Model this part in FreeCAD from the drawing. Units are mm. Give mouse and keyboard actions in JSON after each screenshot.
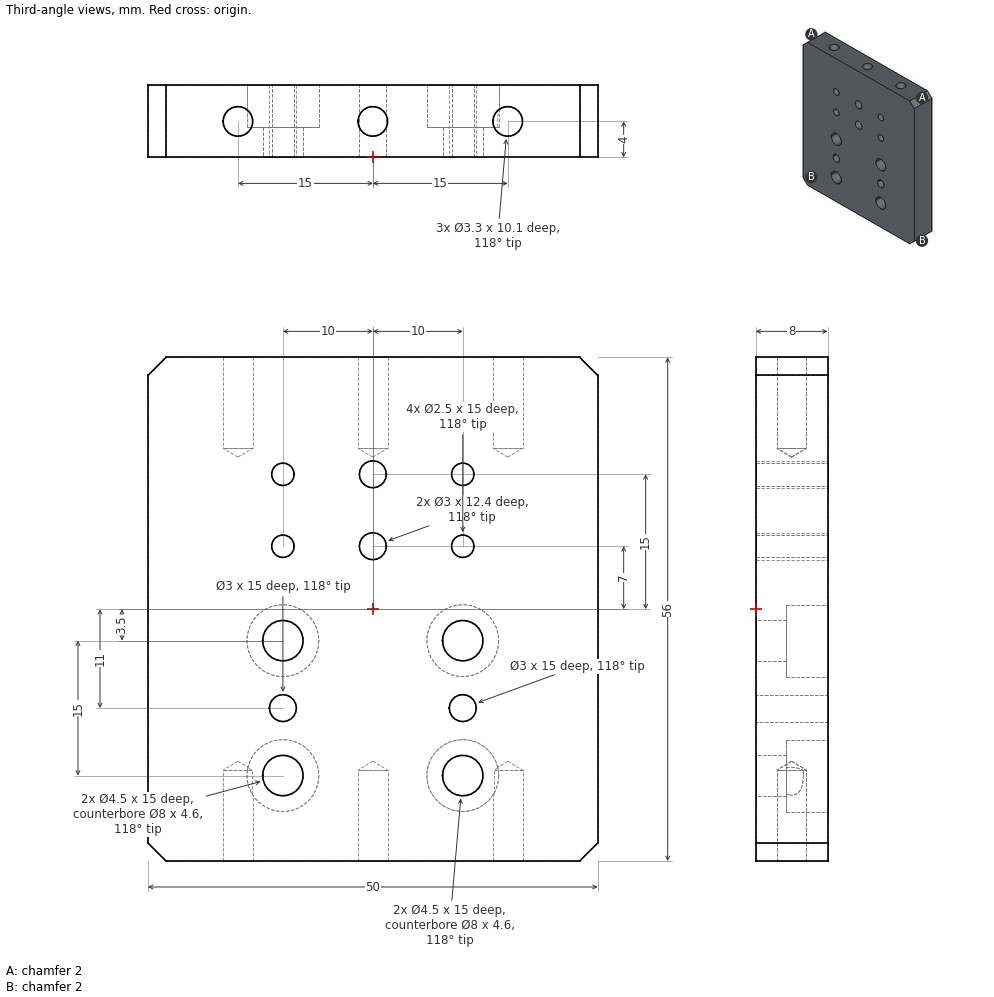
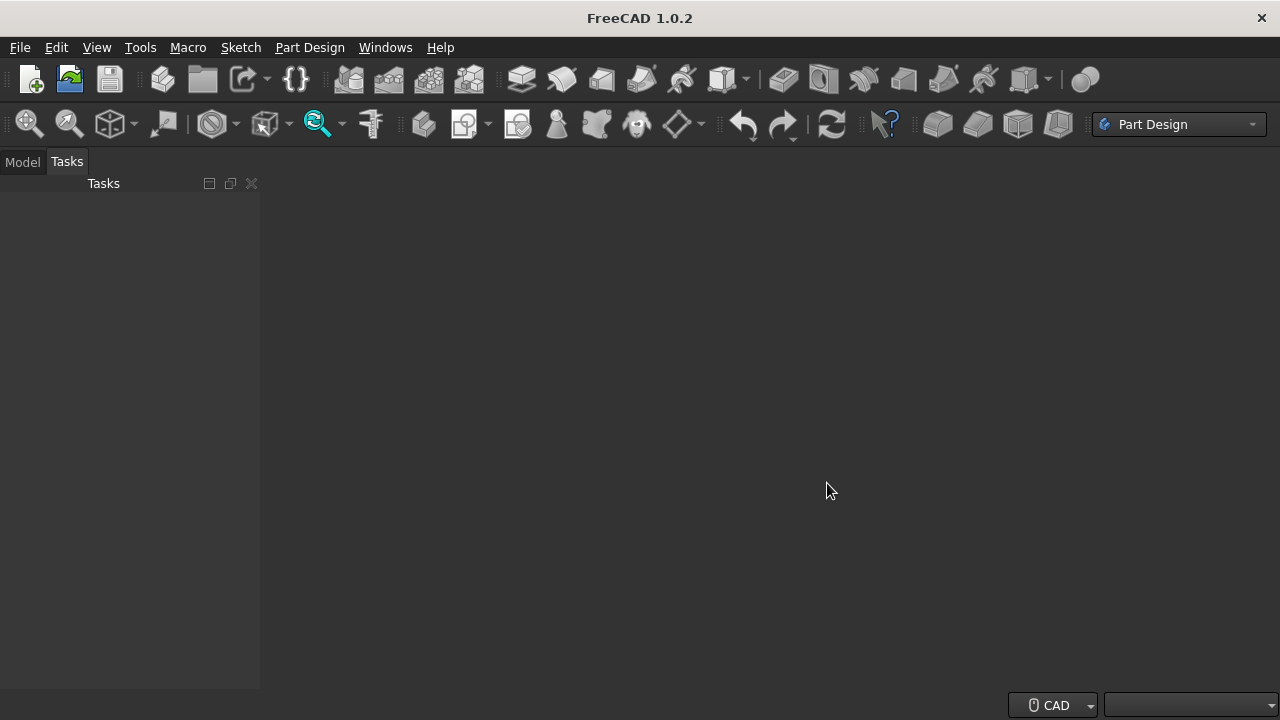
{"action": "left_click", "coordinate": [30, 80]}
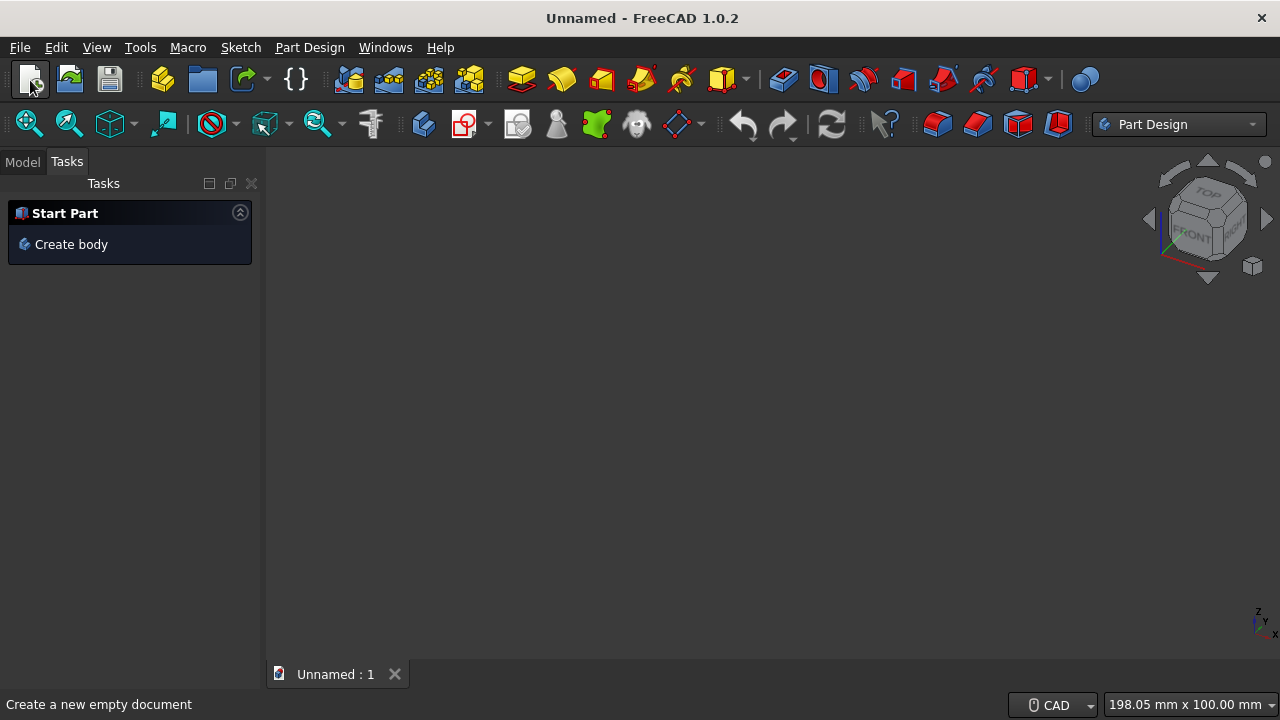
{"action": "left_click", "coordinate": [464, 124]}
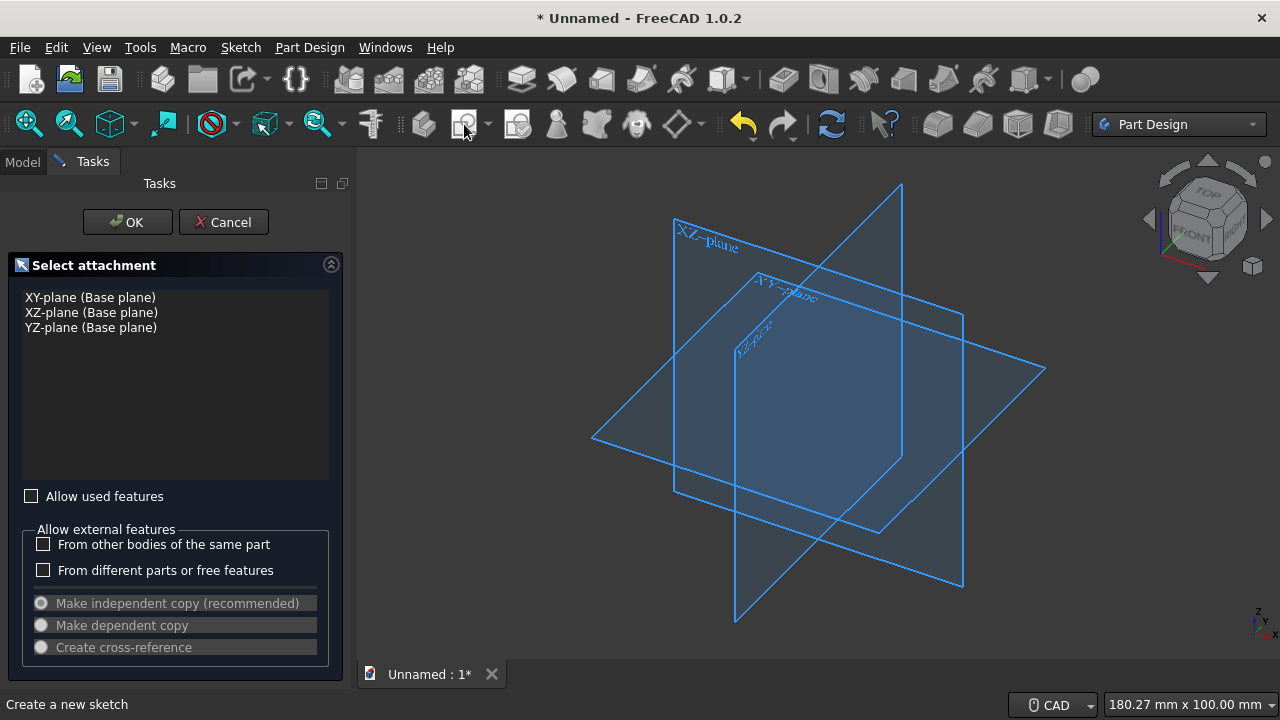
{"action": "left_click", "coordinate": [82, 312]}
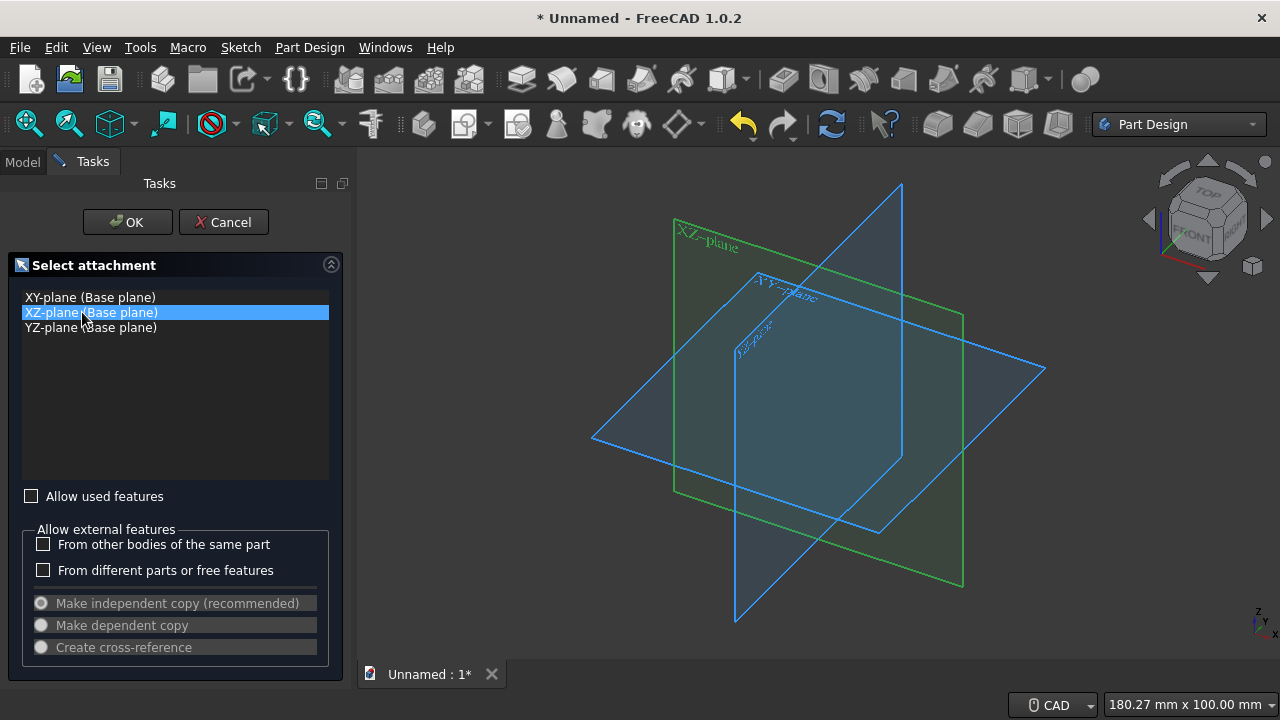
{"action": "left_click", "coordinate": [128, 222]}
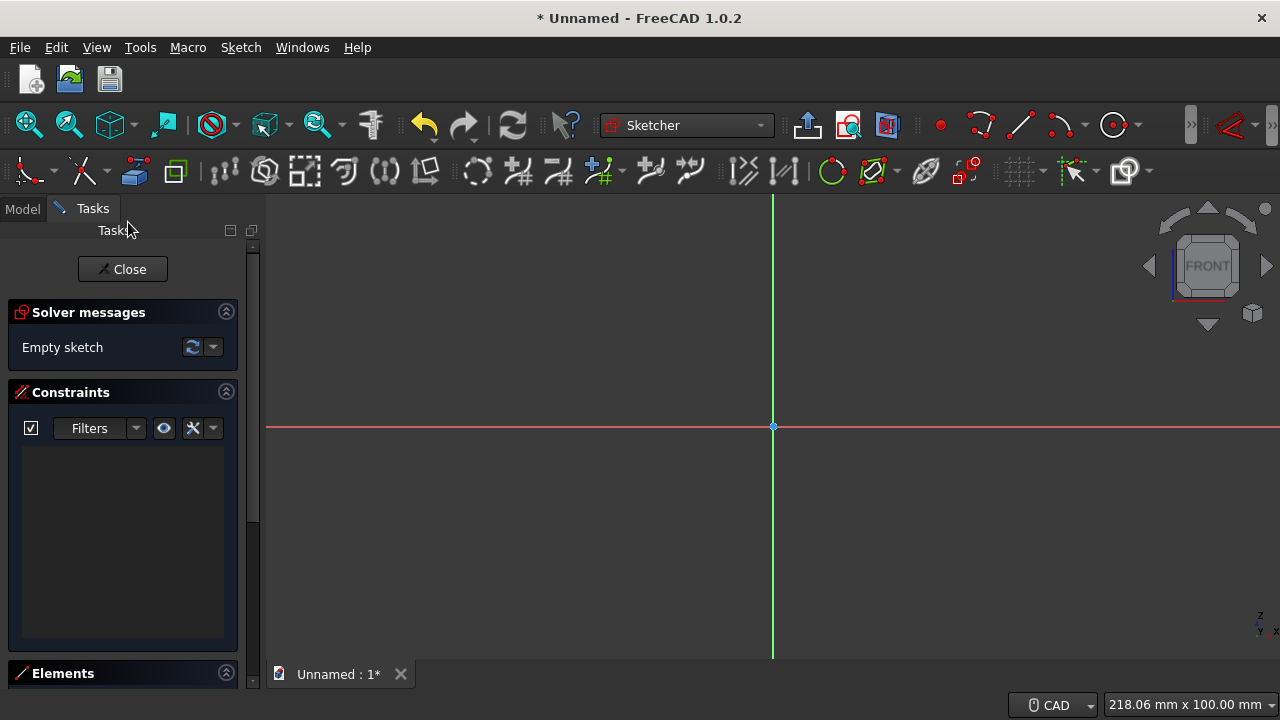
{"action": "key", "text": "g v"}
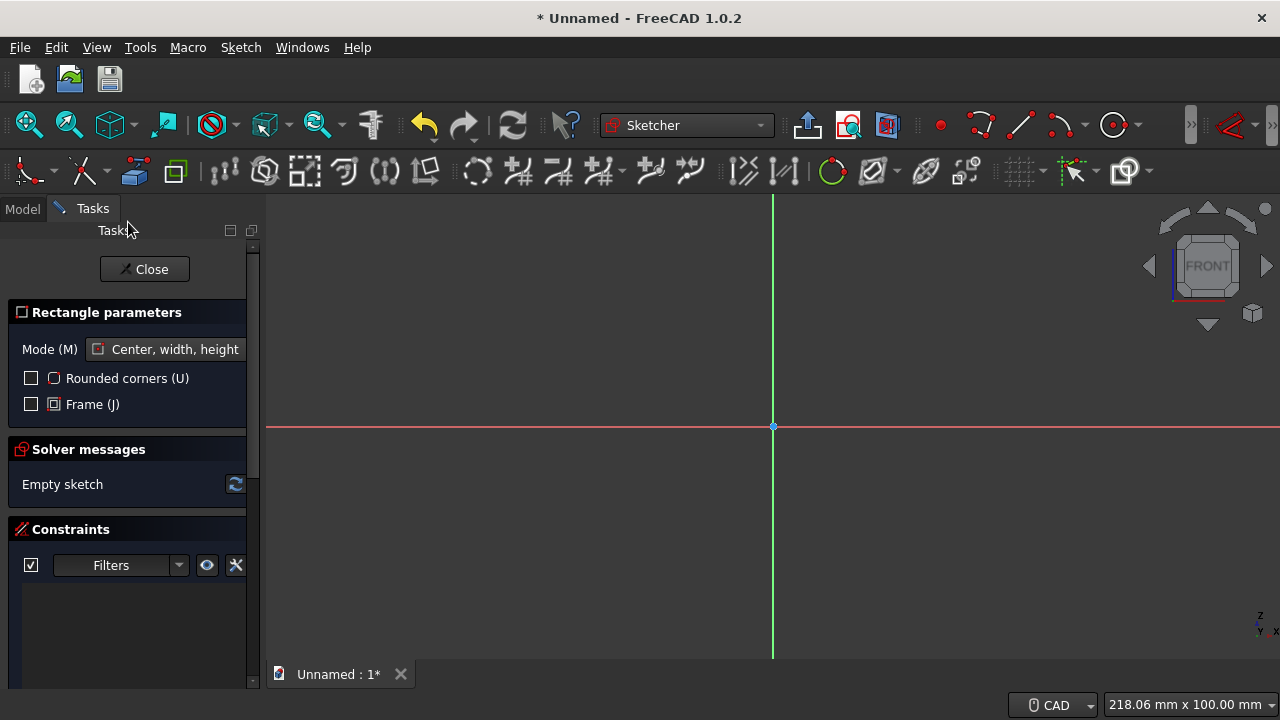
{"action": "left_click", "coordinate": [773, 426]}
{"action": "mouse_move", "coordinate": [889, 296]}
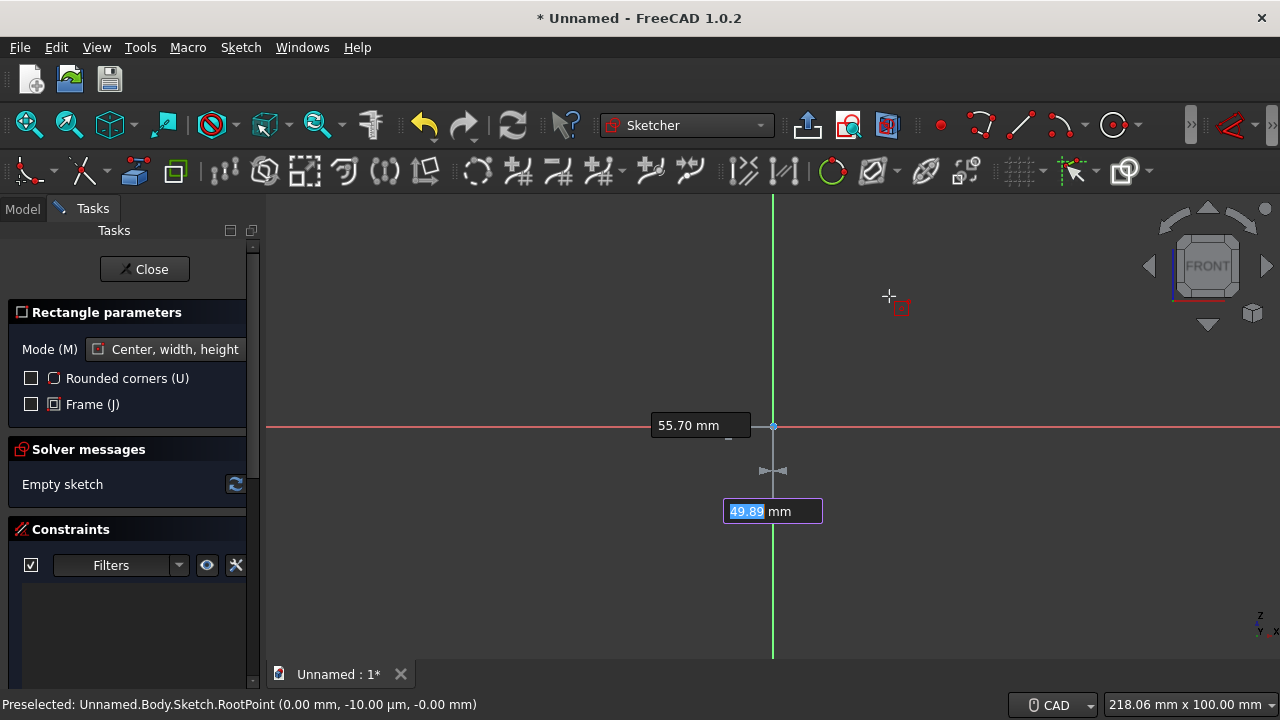
{"action": "type", "text": "50"}
{"action": "key", "text": "Tab"}
{"action": "type", "text": "56"}
{"action": "key", "text": "Return"}
{"action": "key", "text": "Escape"}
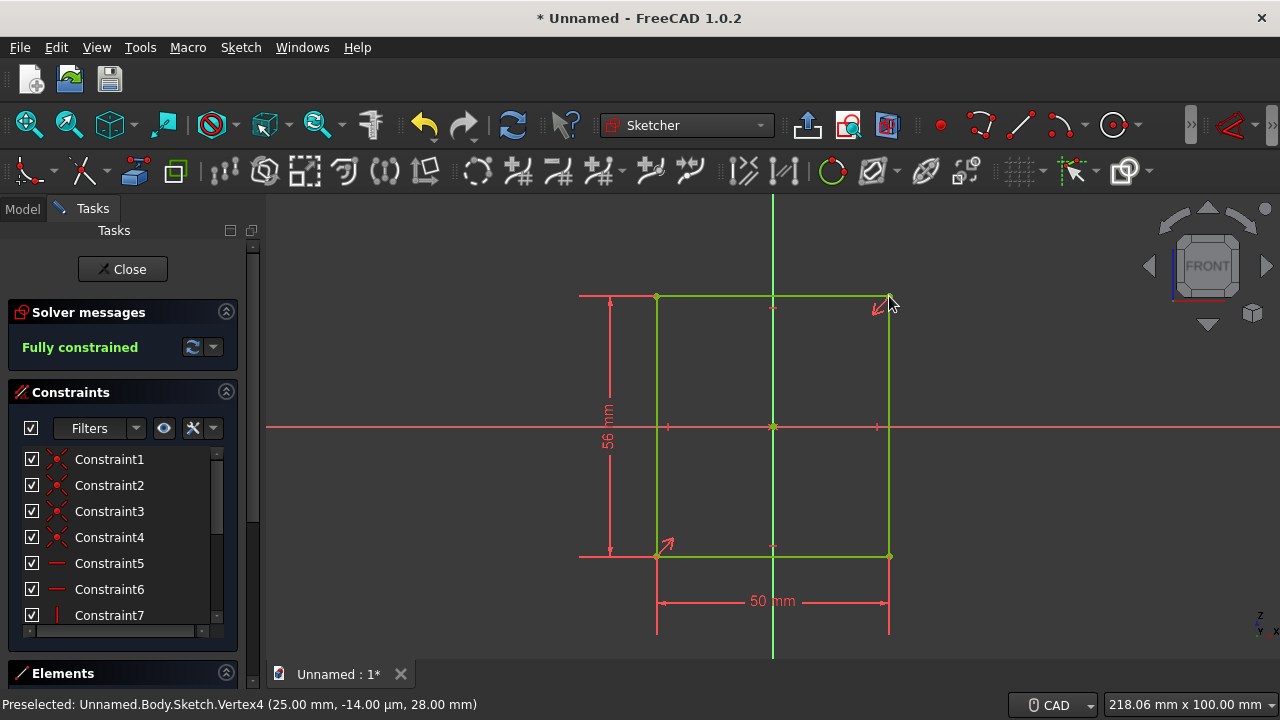
{"action": "left_click", "coordinate": [123, 269]}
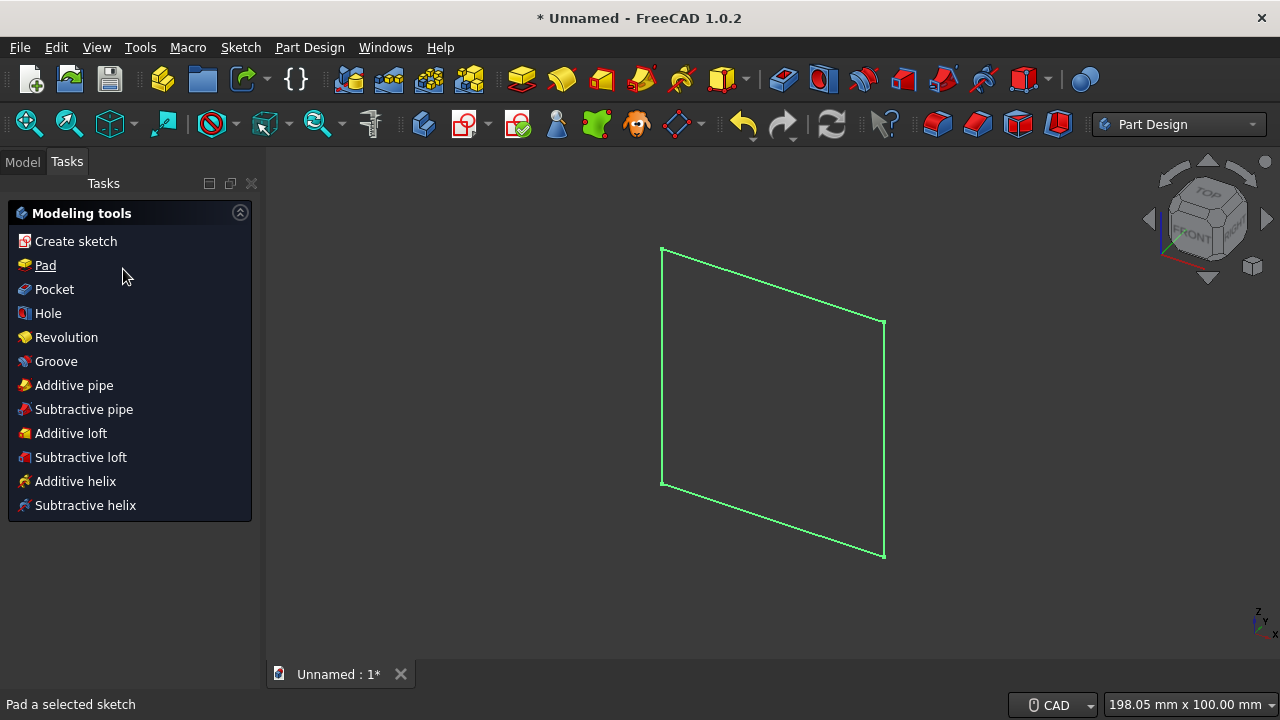
{"action": "left_click", "coordinate": [522, 80]}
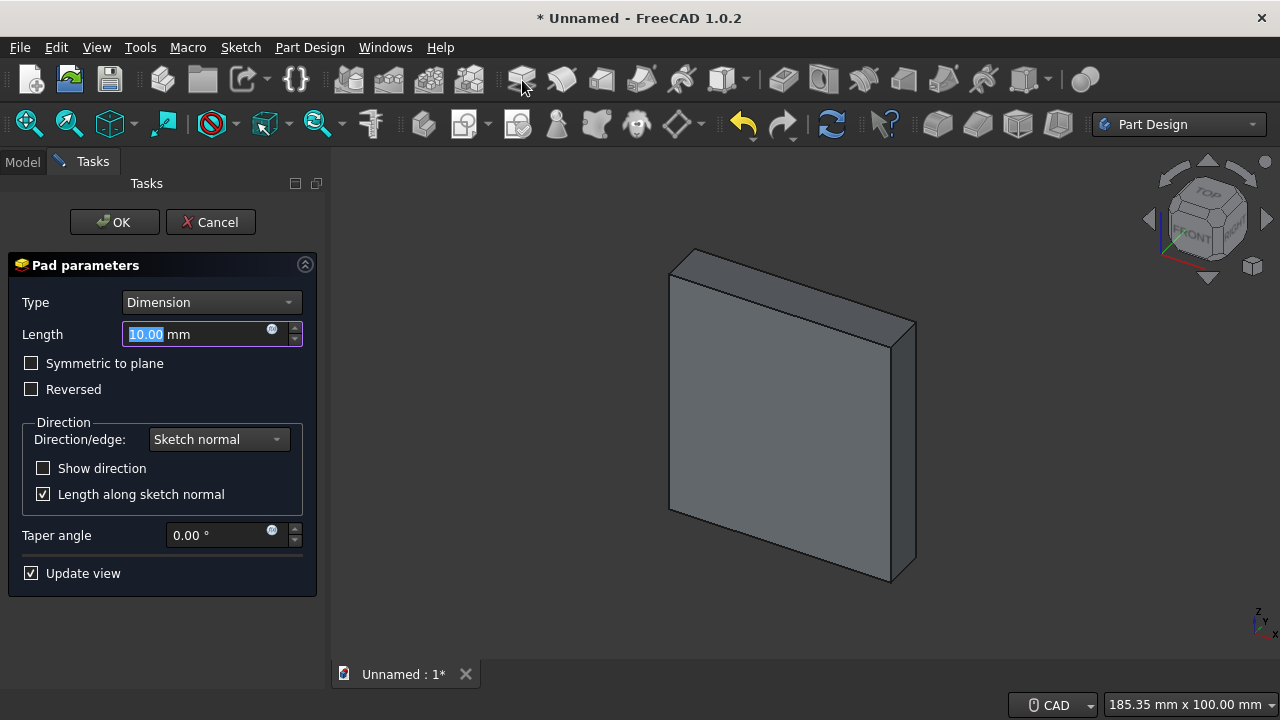
{"action": "type", "text": "8"}
{"action": "key", "text": "Tab"}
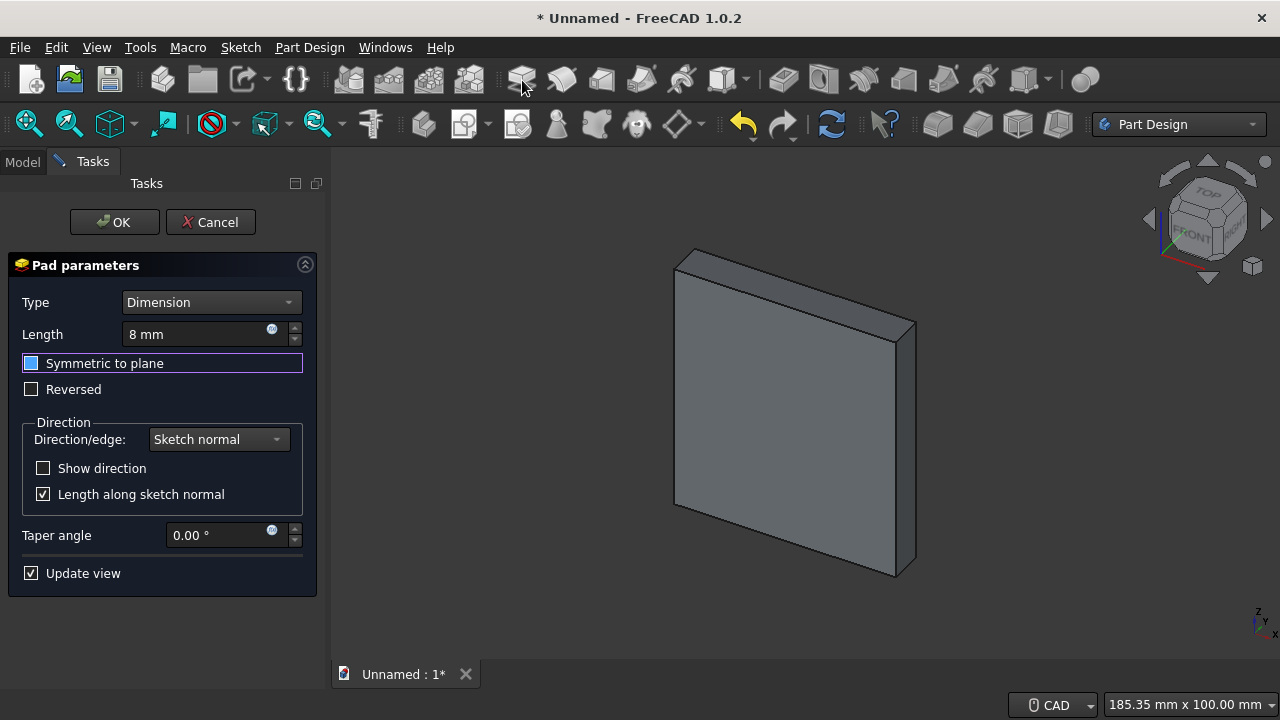
{"action": "left_click", "coordinate": [30, 389]}